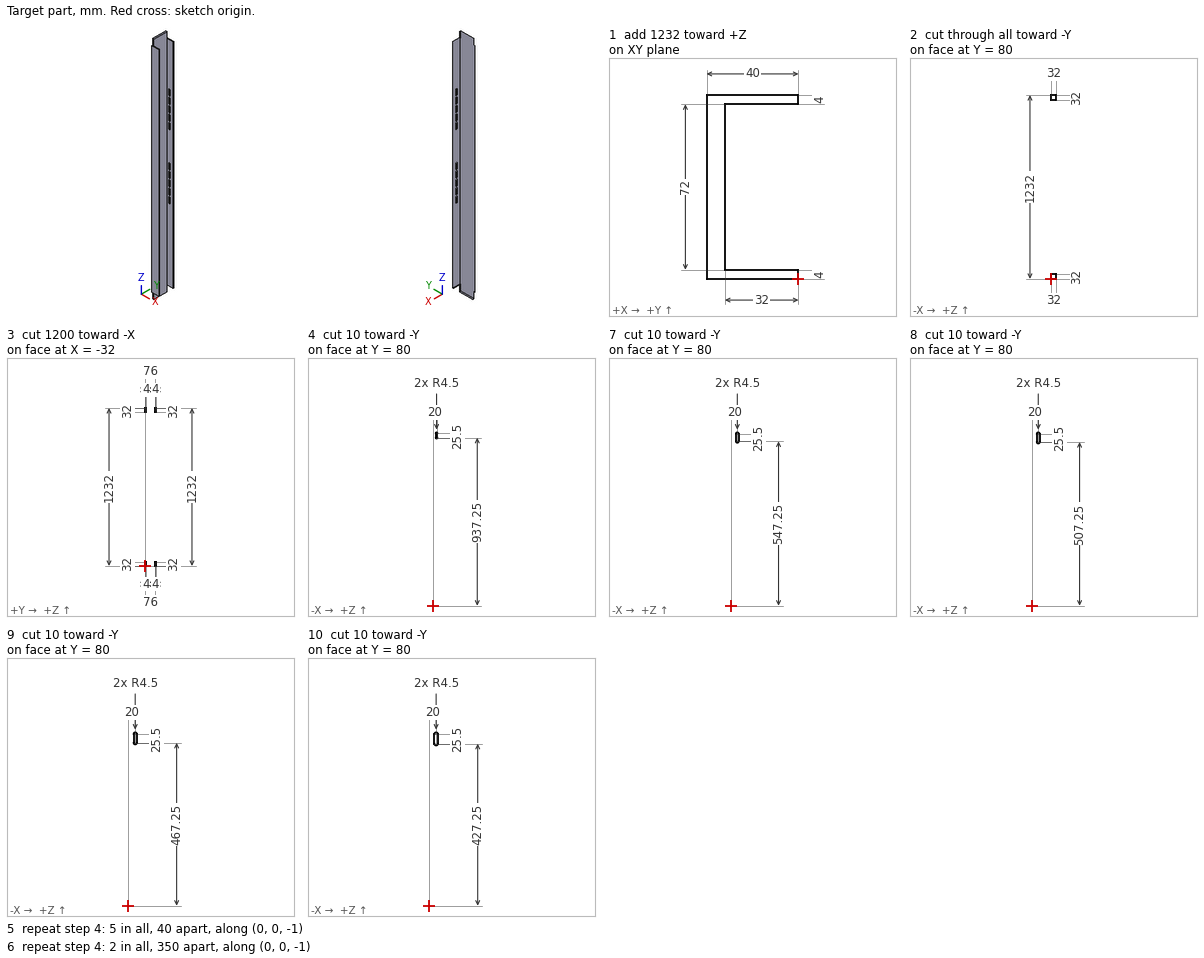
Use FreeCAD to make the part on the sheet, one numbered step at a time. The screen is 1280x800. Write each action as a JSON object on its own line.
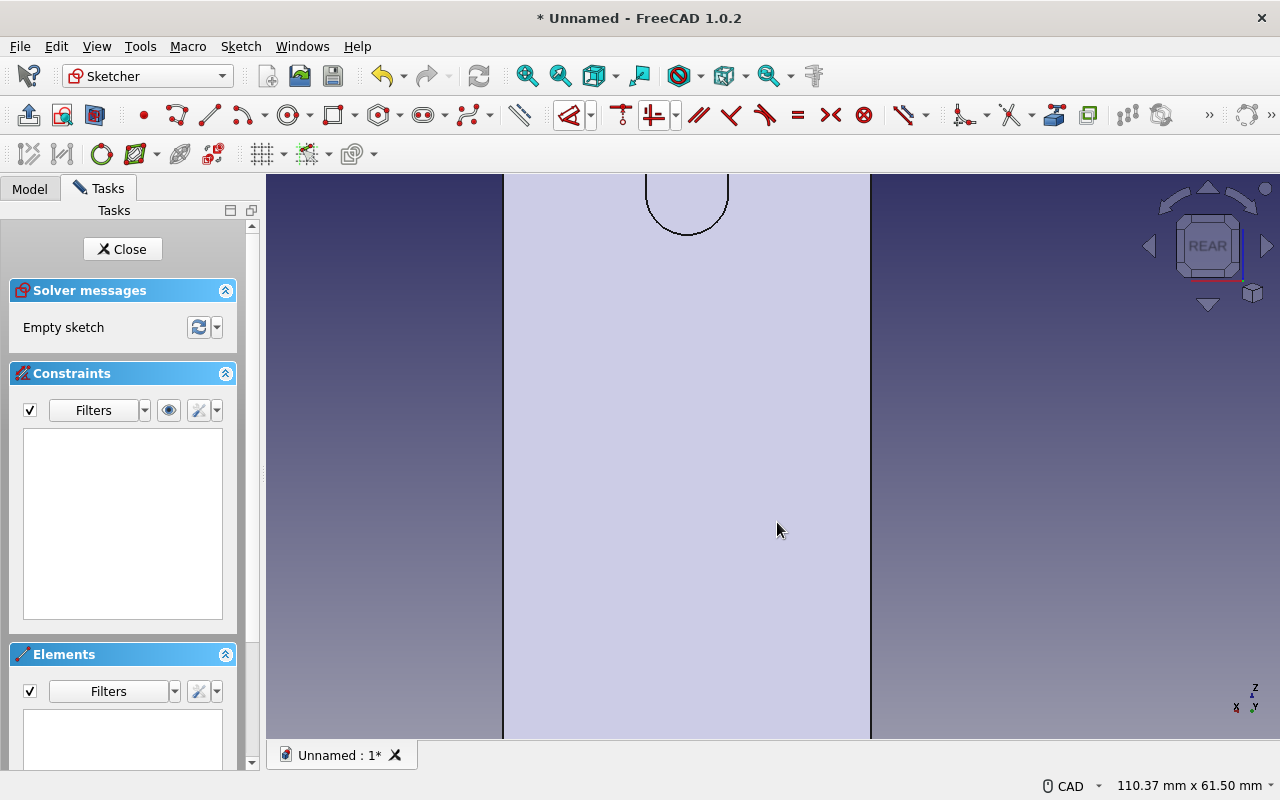
{"action": "left_click", "coordinate": [422, 116]}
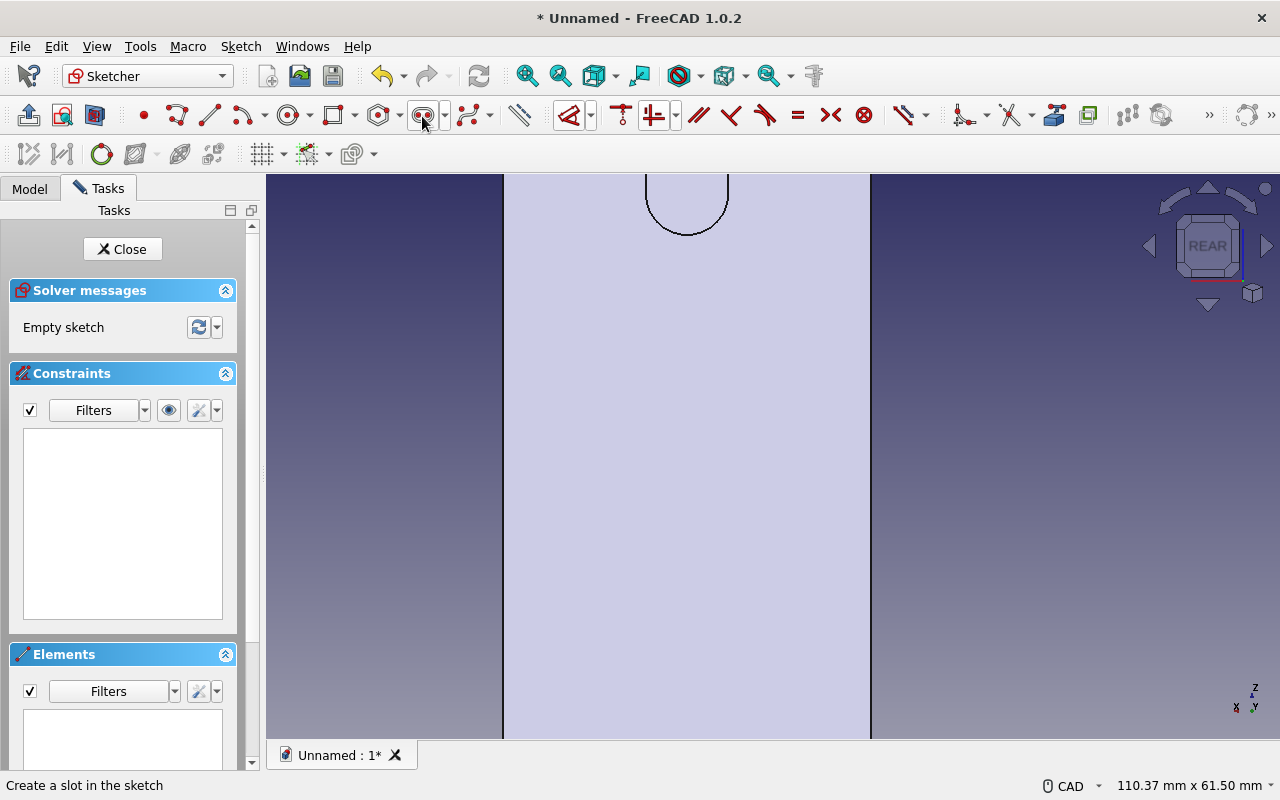
{"action": "left_click", "coordinate": [687, 561]}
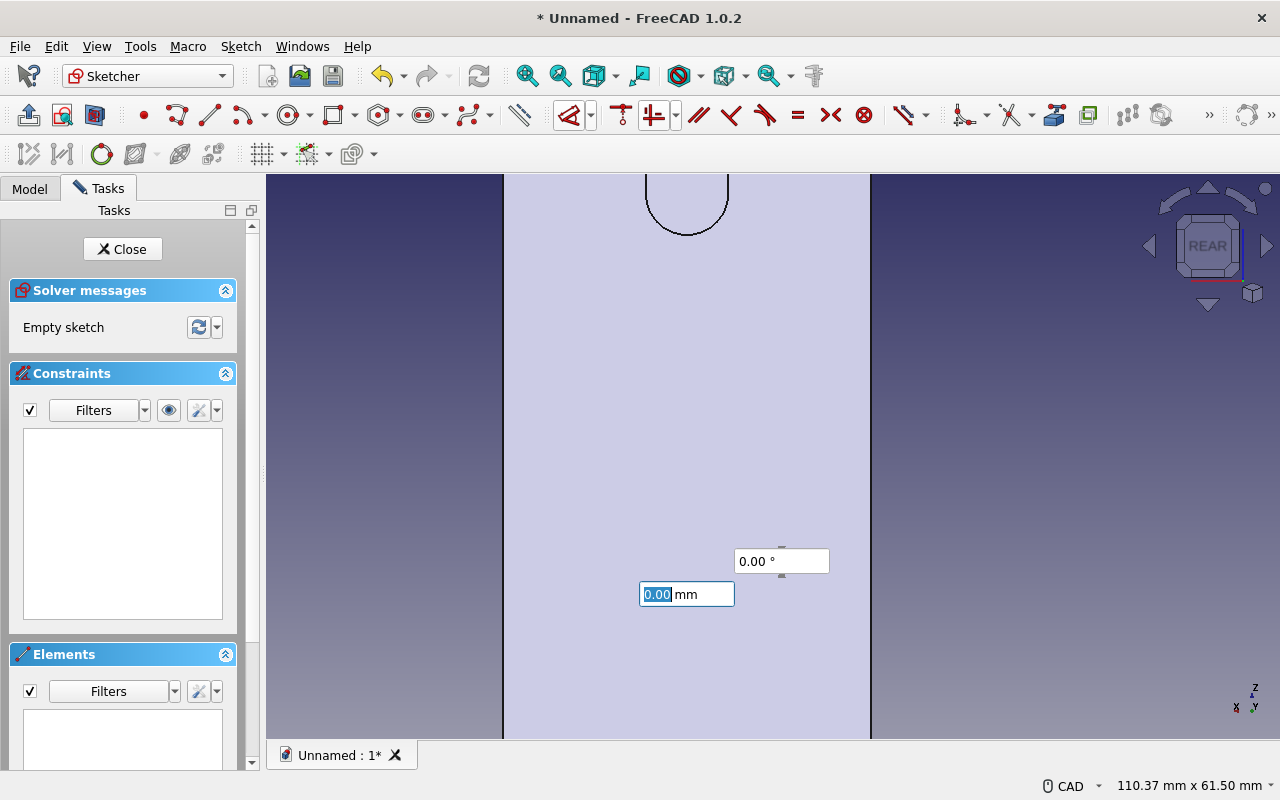
{"action": "left_click", "coordinate": [687, 327]}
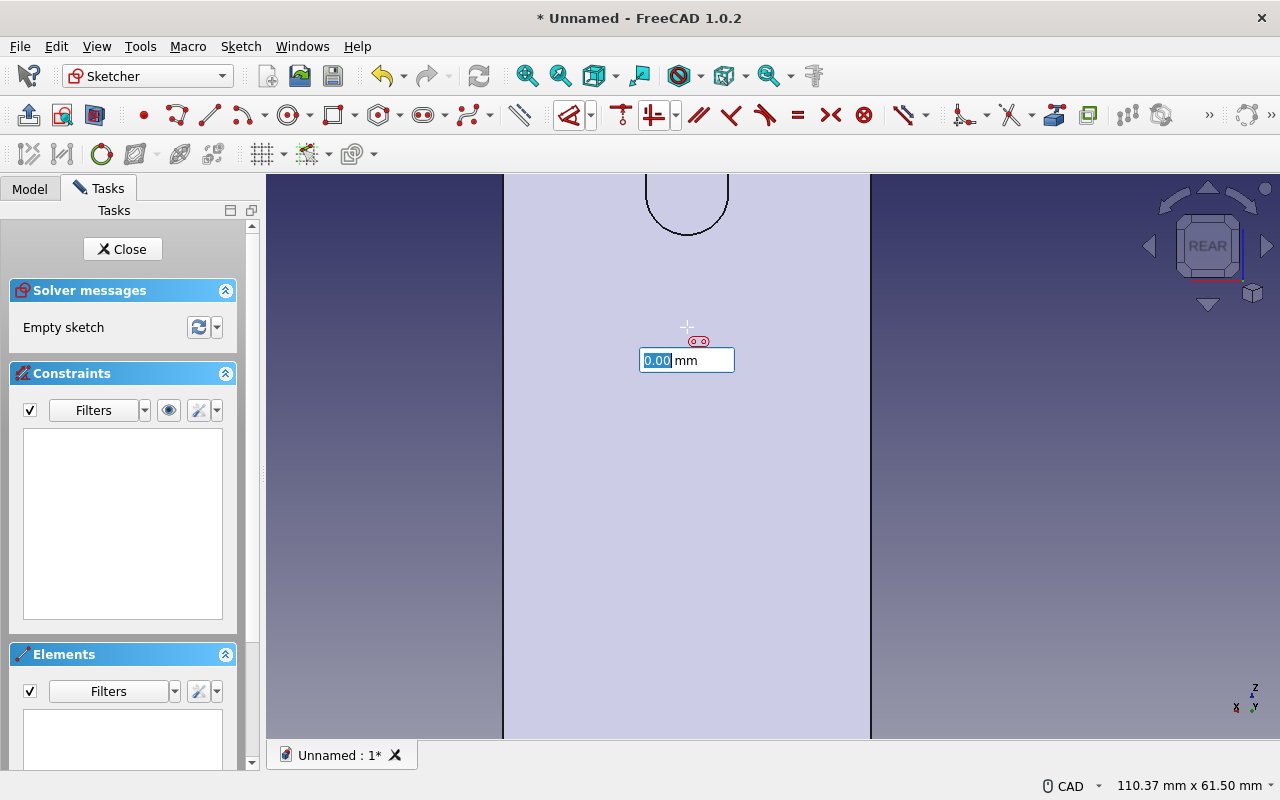
{"action": "left_click", "coordinate": [728, 444]}
{"action": "key", "text": "Escape"}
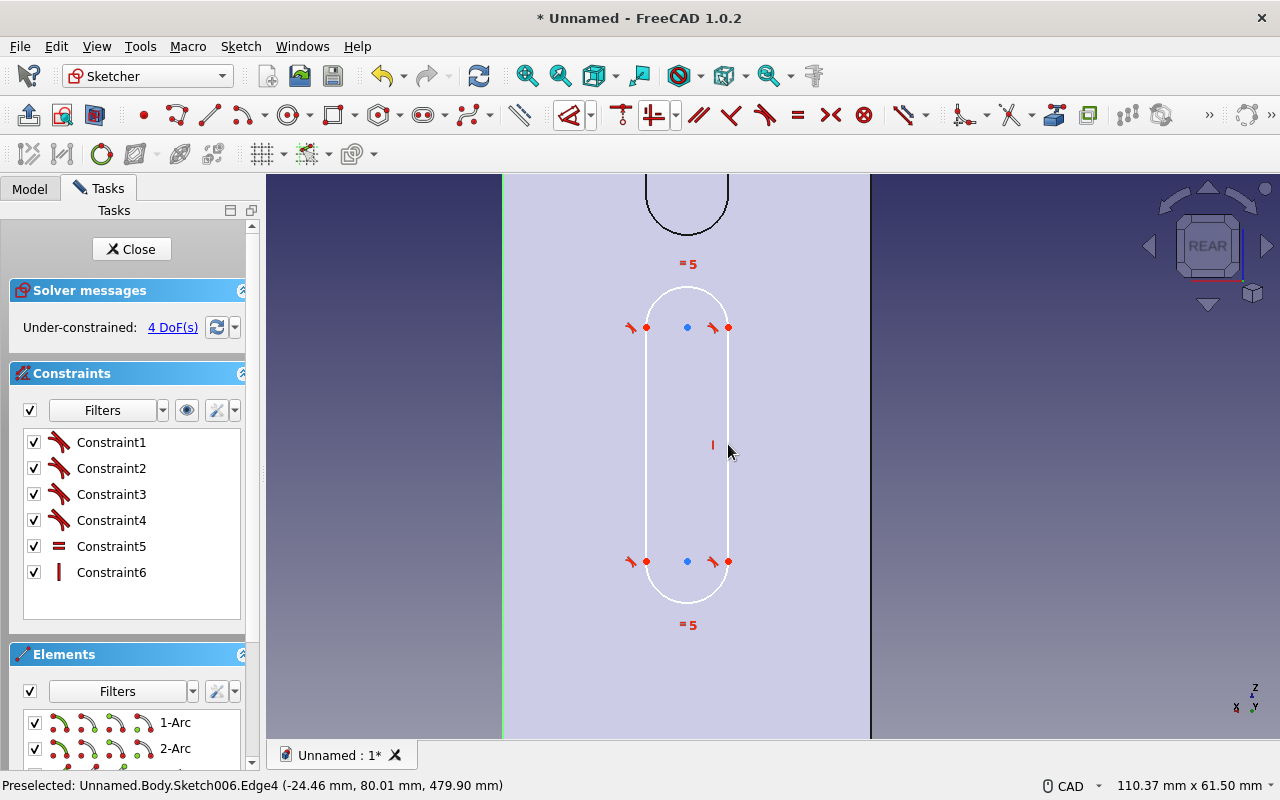
{"action": "left_click", "coordinate": [663, 595]}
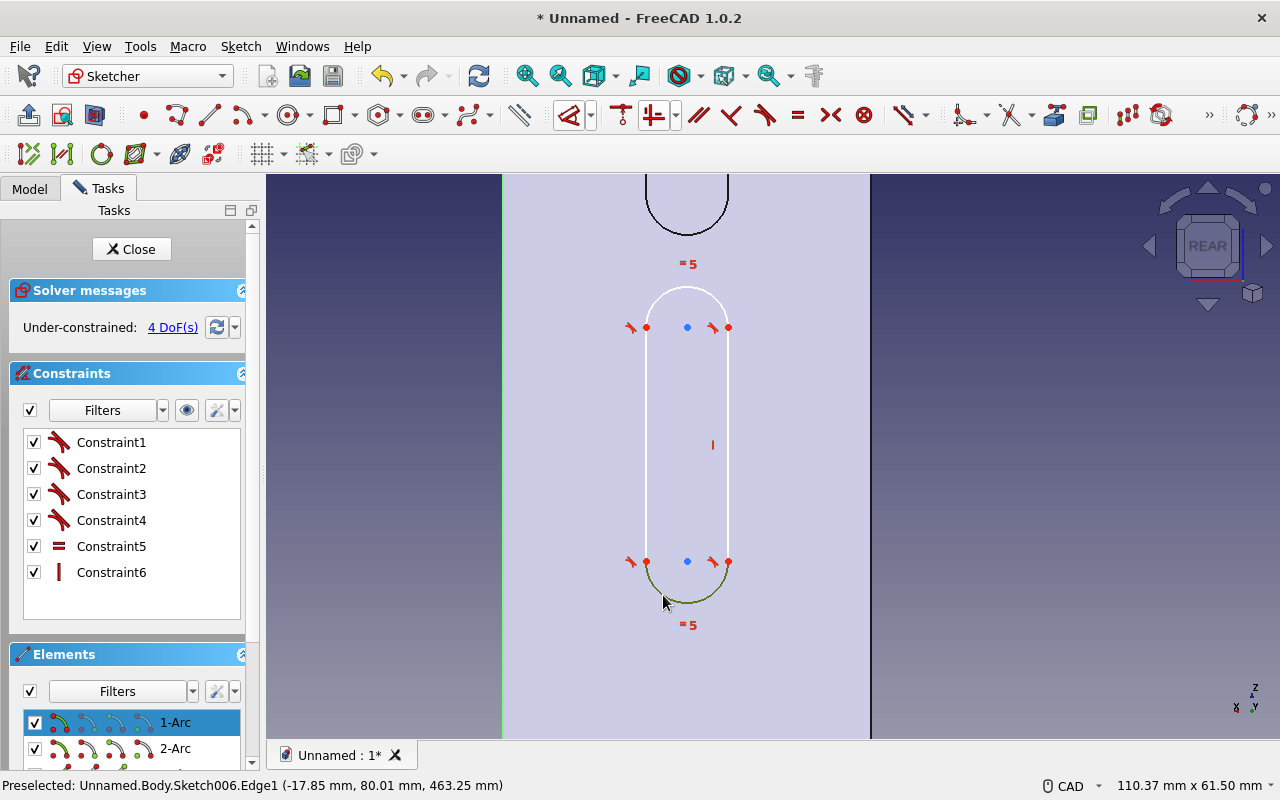
{"action": "left_click", "coordinate": [590, 116]}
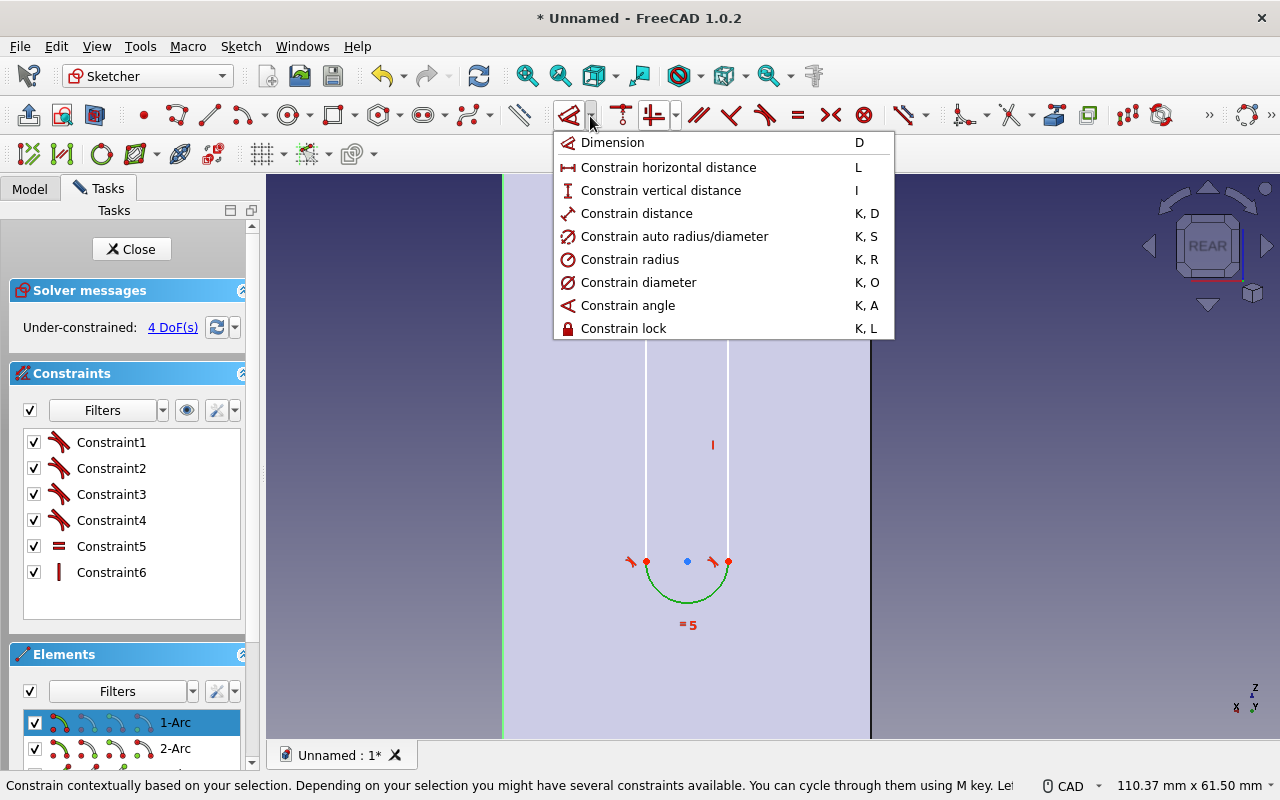
{"action": "left_click", "coordinate": [724, 260]}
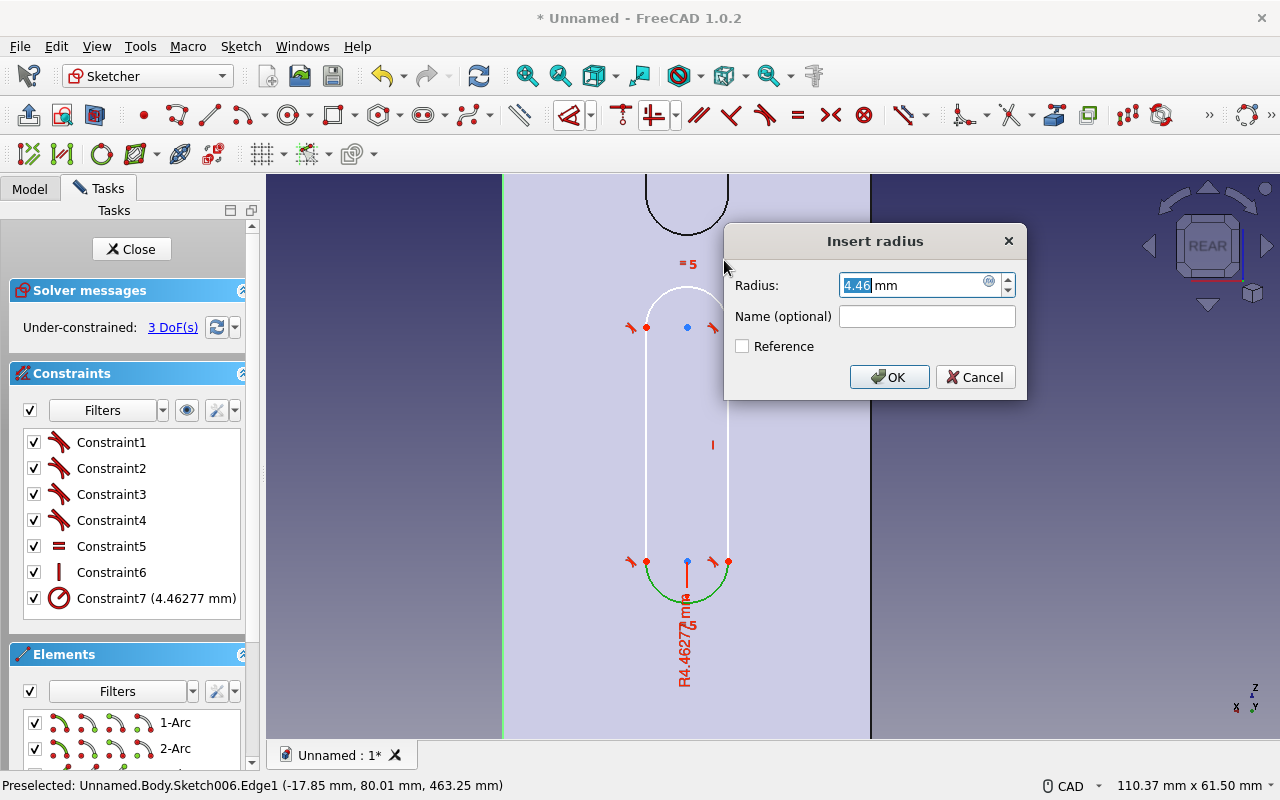
{"action": "type", "text": "4.5"}
{"action": "key", "text": "Return"}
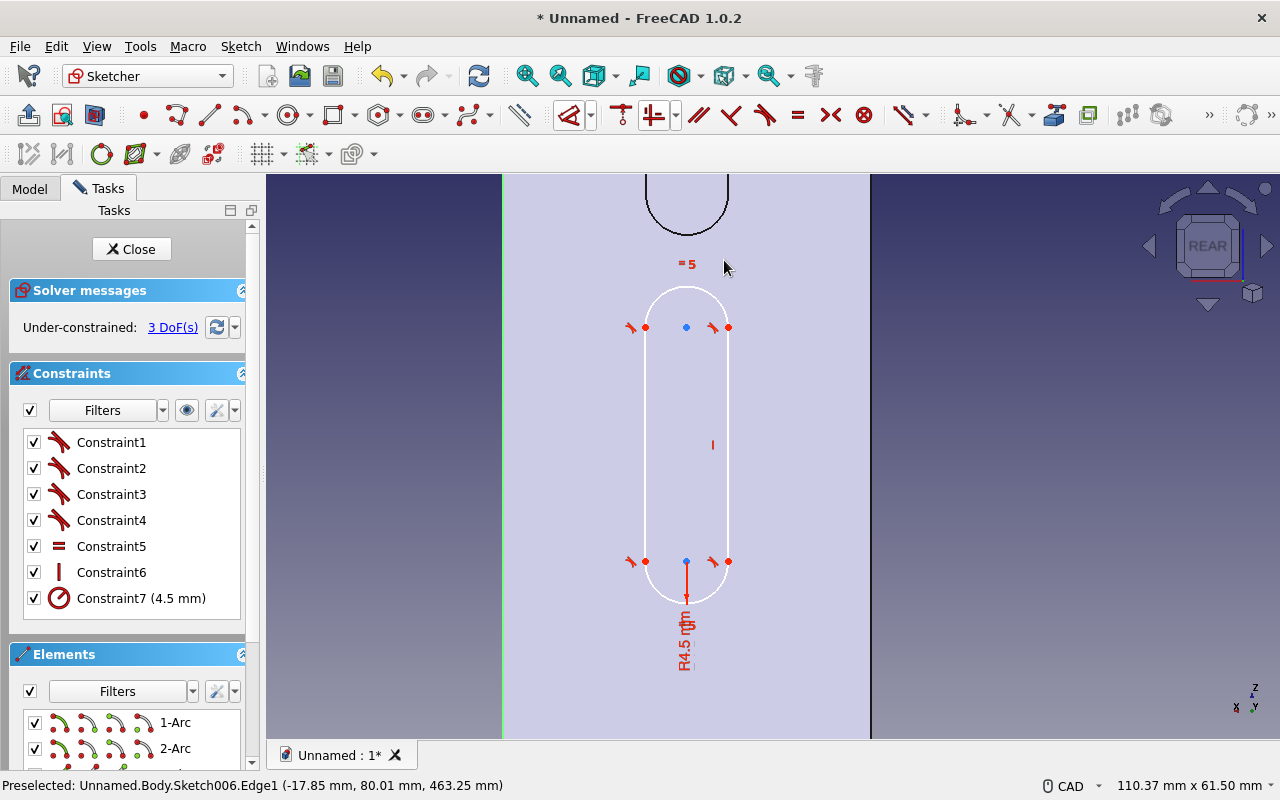
{"action": "left_click", "coordinate": [687, 562]}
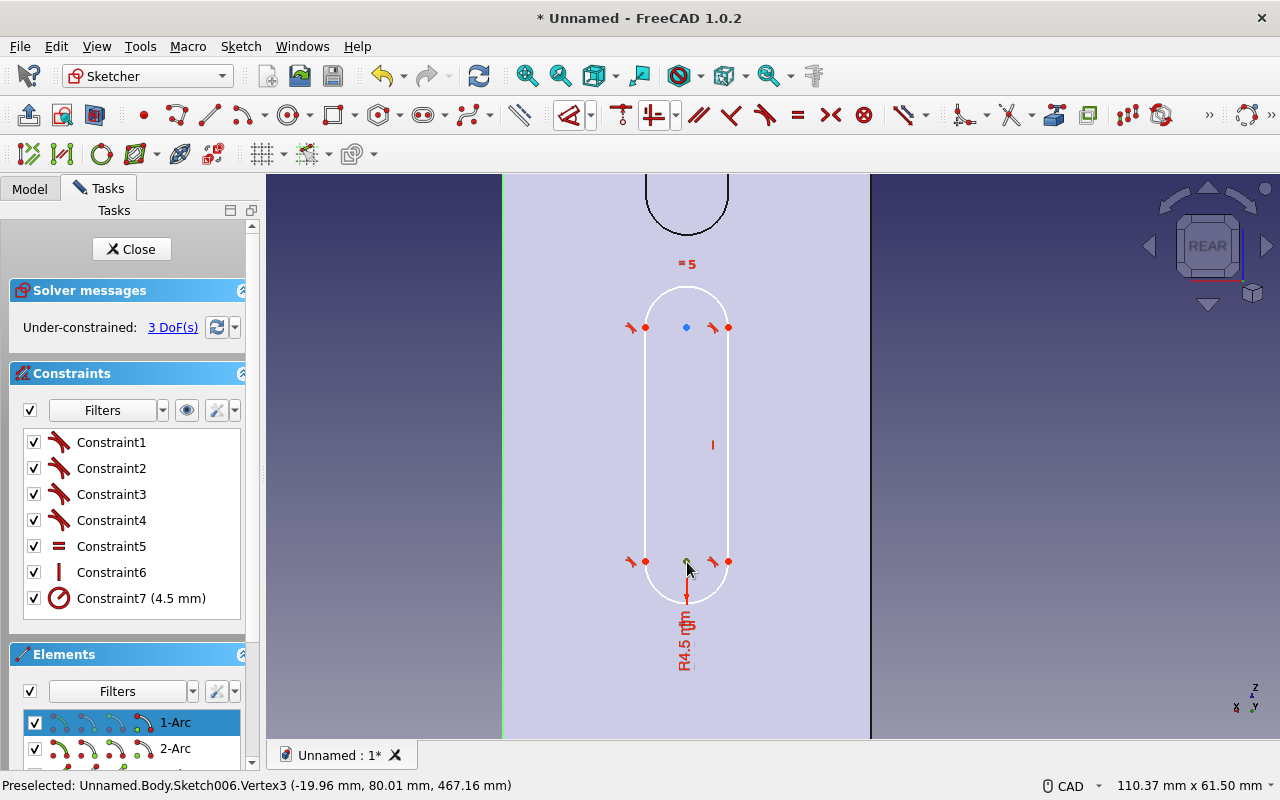
{"action": "key", "text": "l"}